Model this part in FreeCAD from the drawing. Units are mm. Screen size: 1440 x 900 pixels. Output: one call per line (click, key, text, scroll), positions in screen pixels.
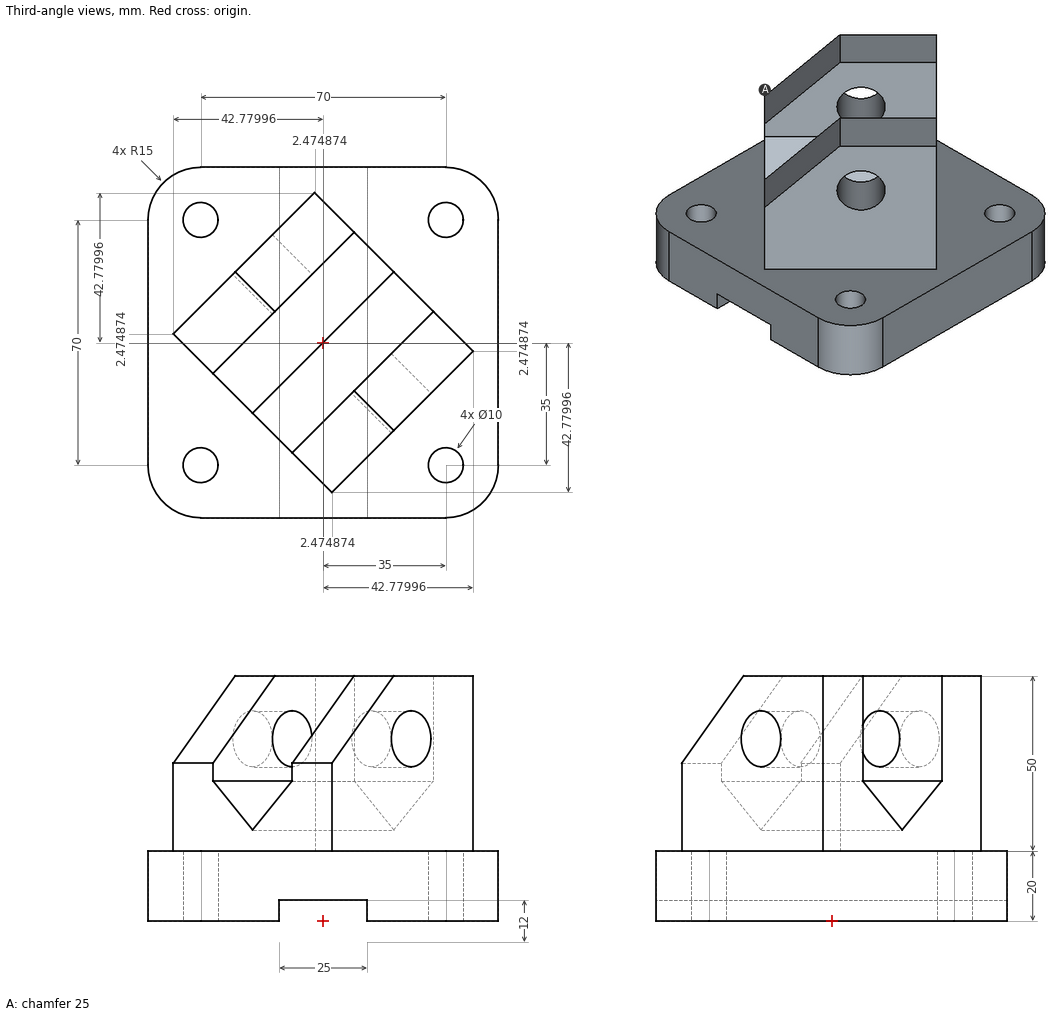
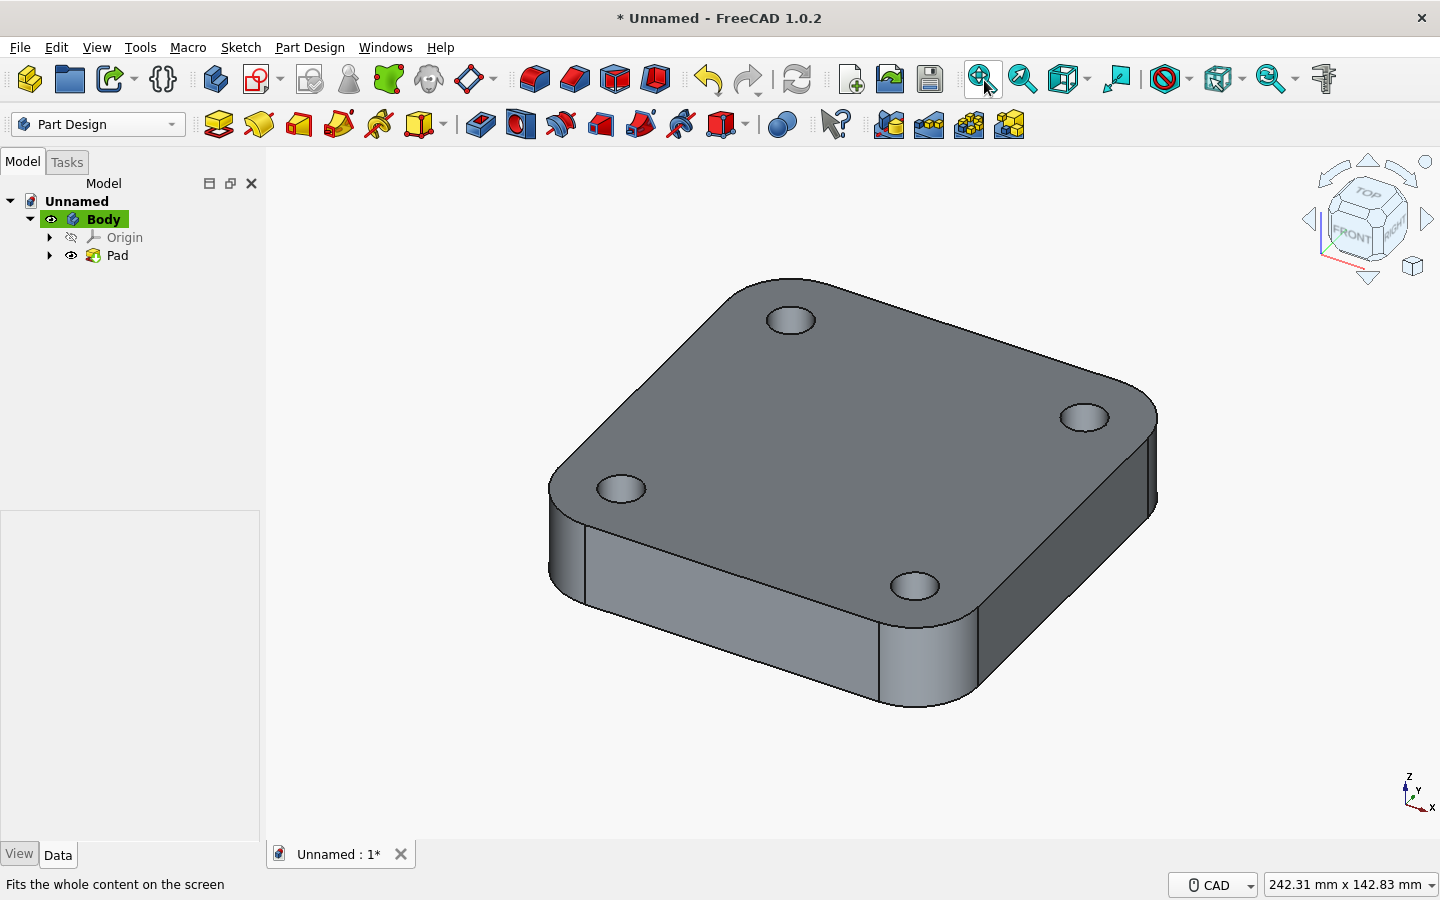
click(816, 640)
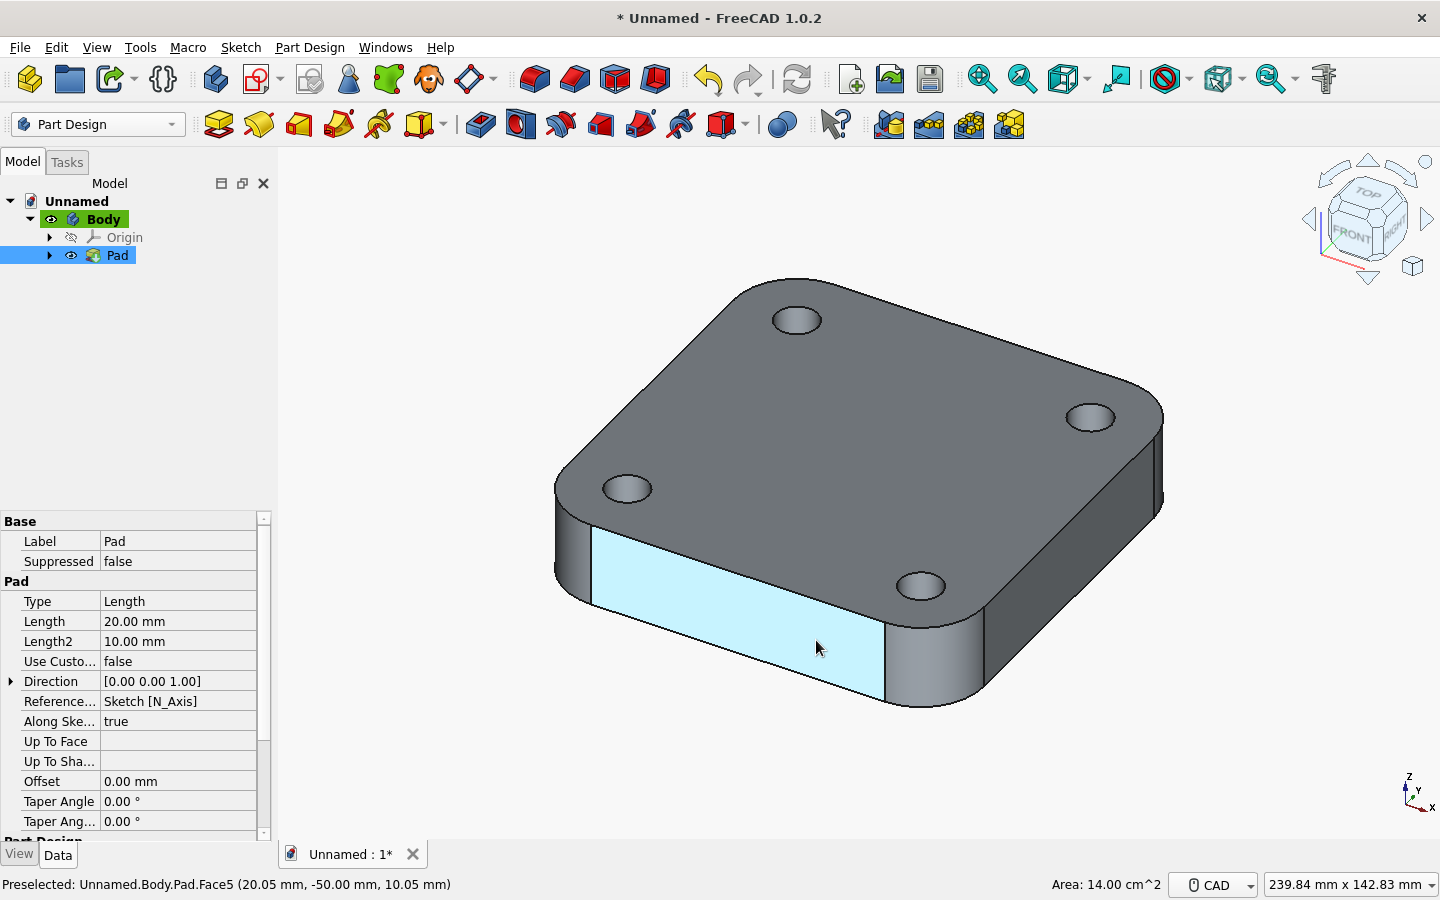
click(256, 80)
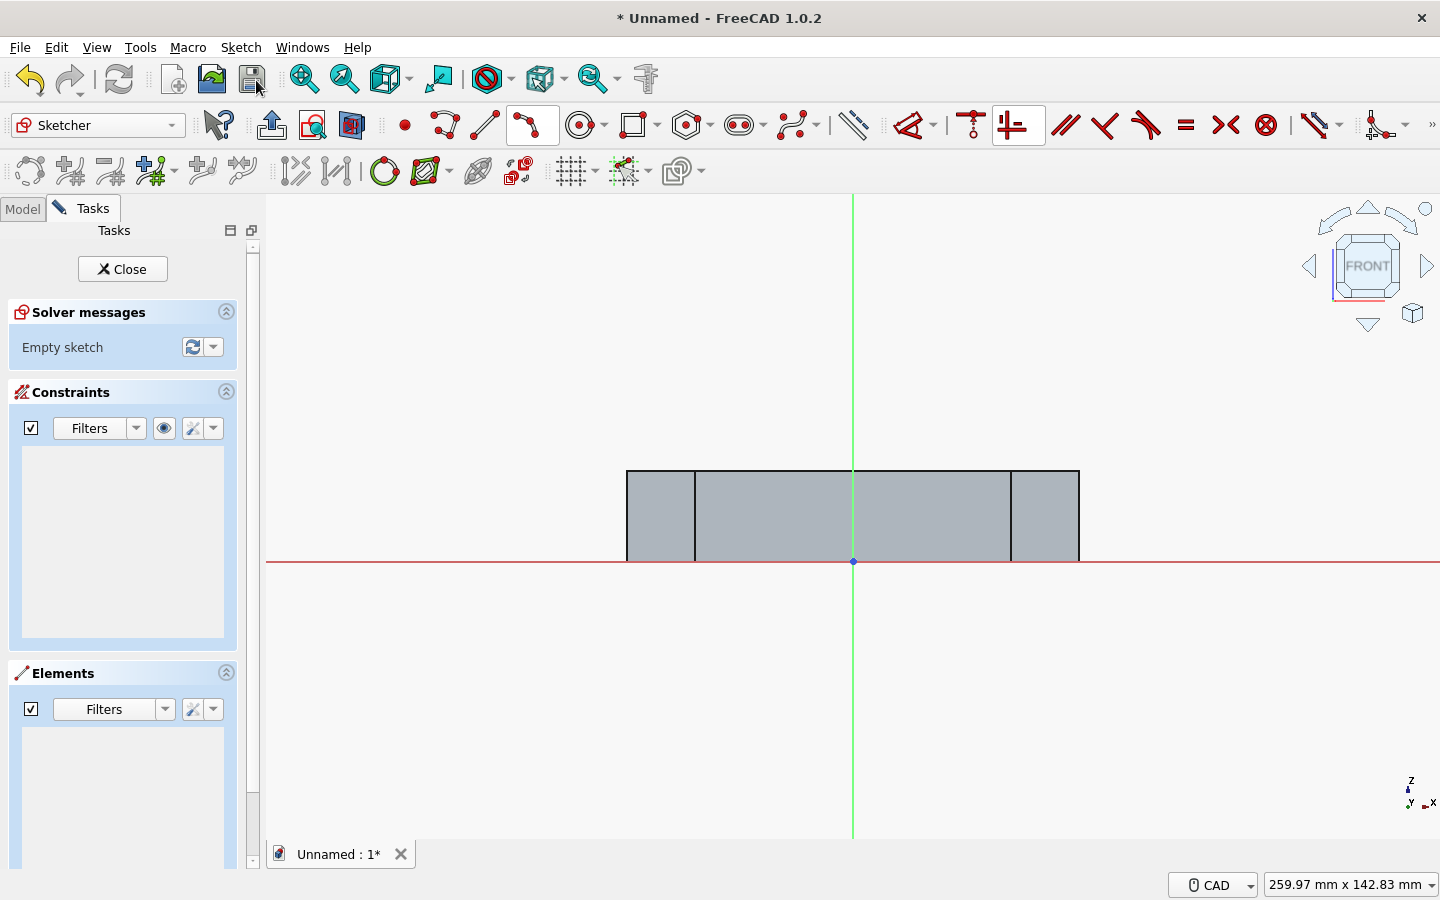
scroll(867, 571, up, 9)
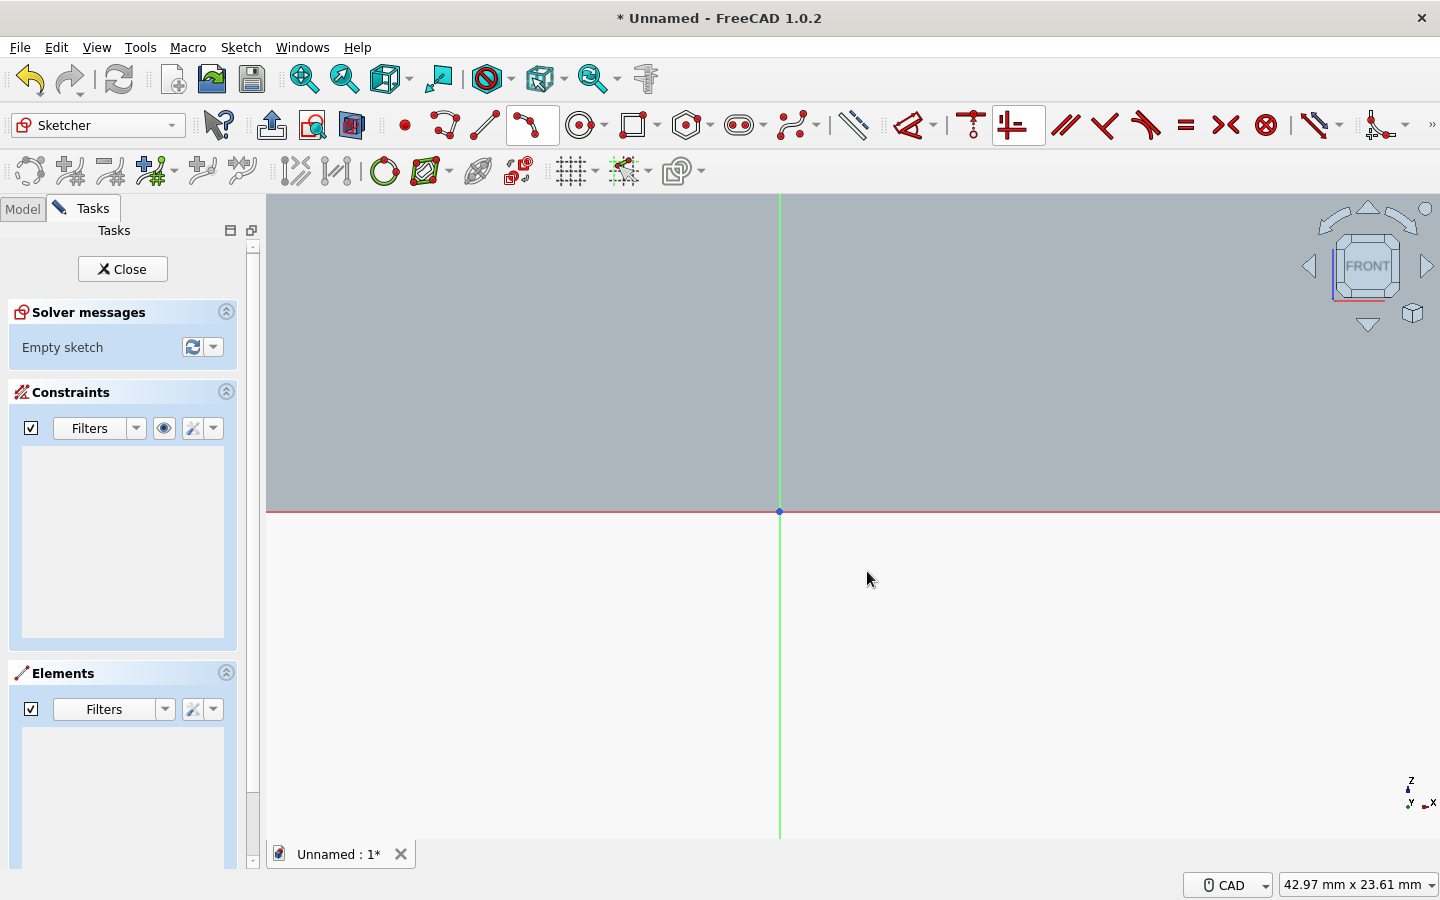
key(g)
key(v)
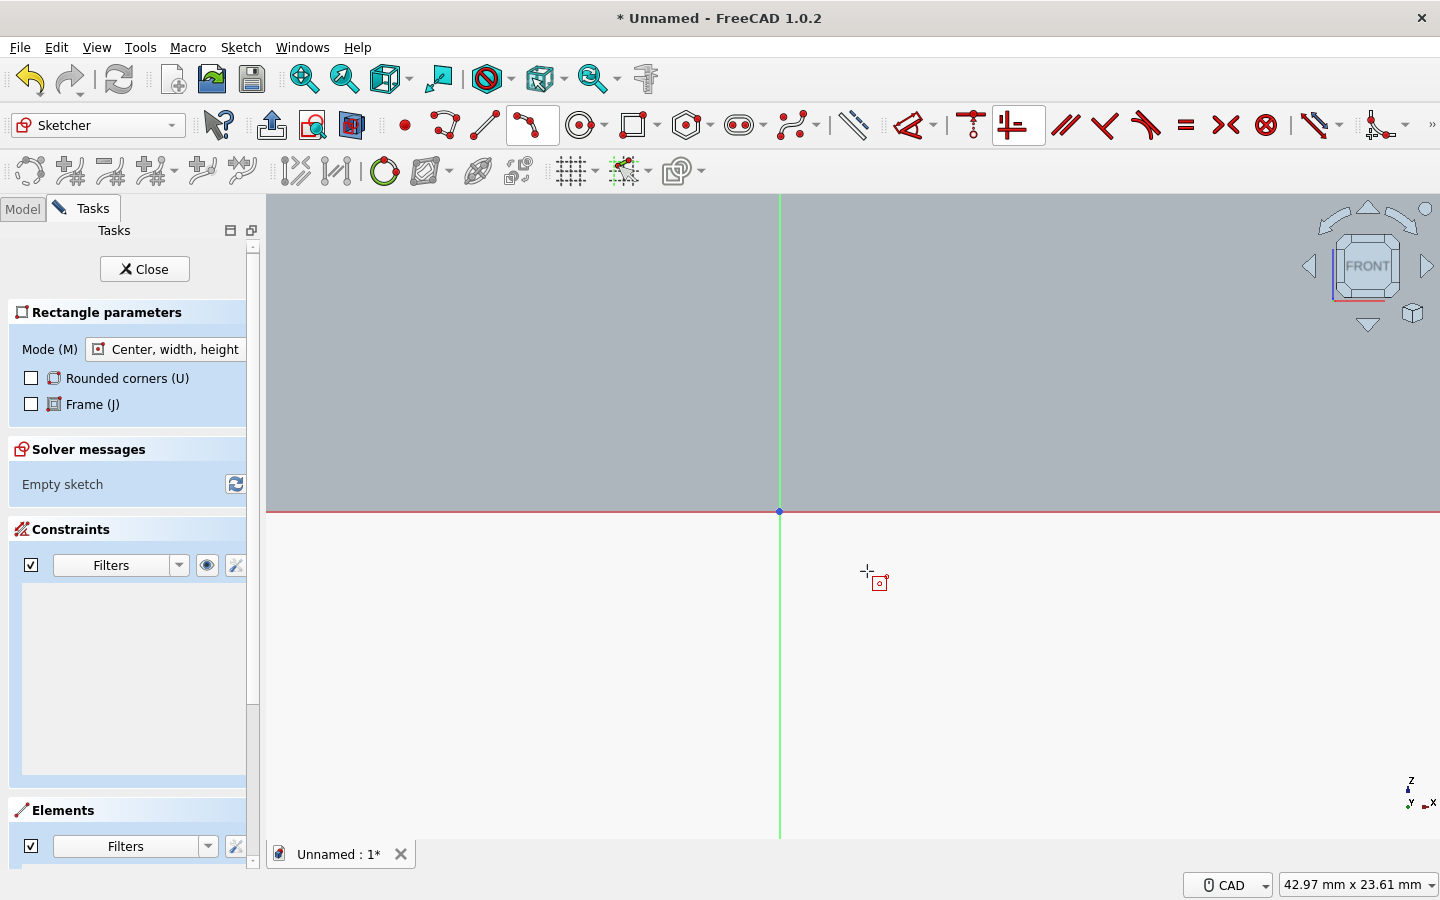
click(780, 512)
move(1121, 348)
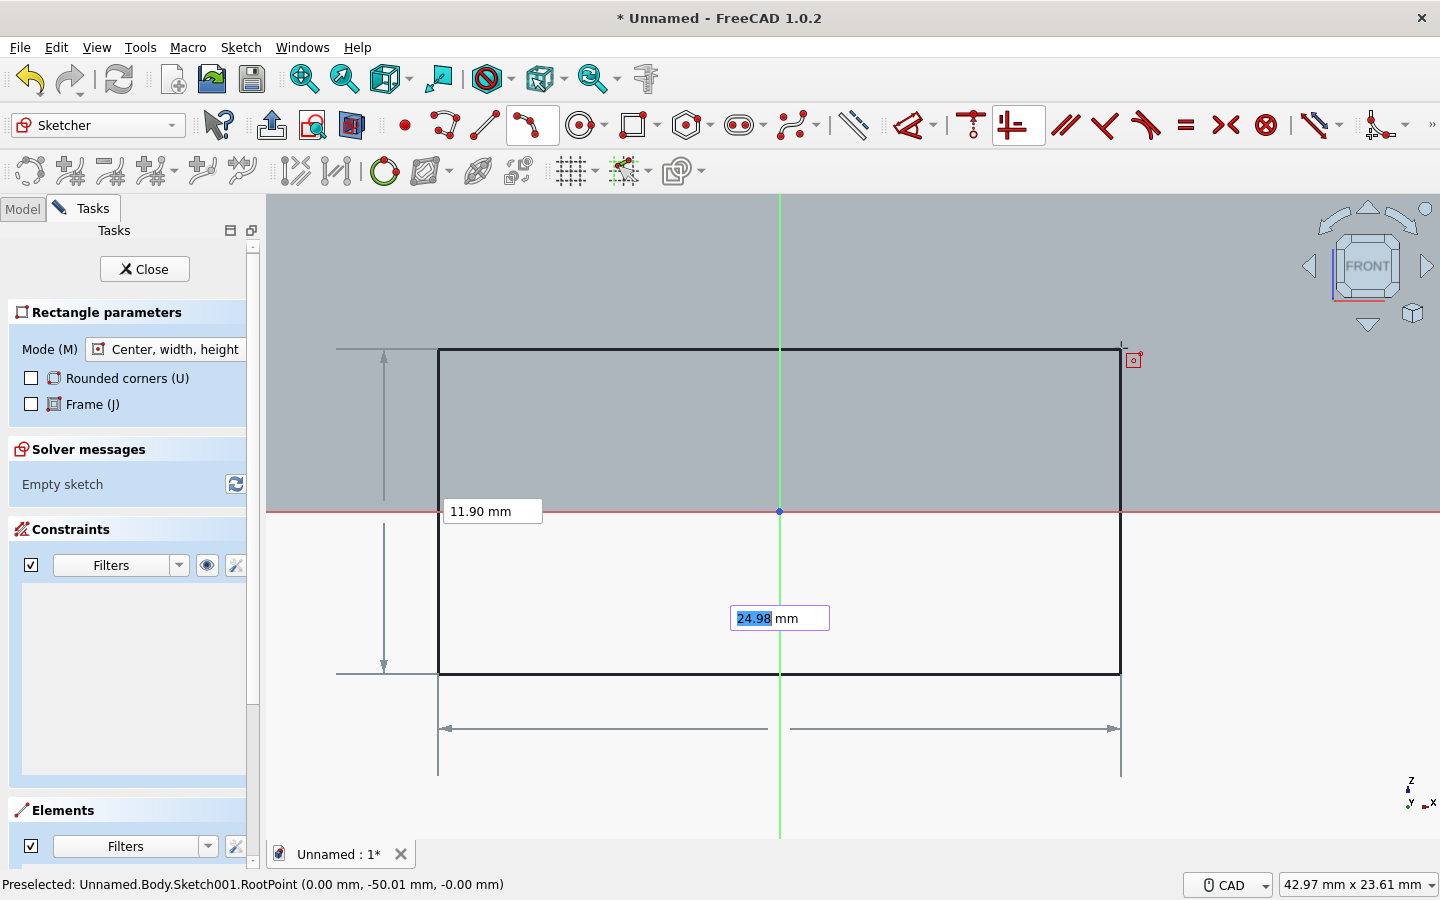
text(25)
key(Tab)
text(12)
key(Return)
key(Escape)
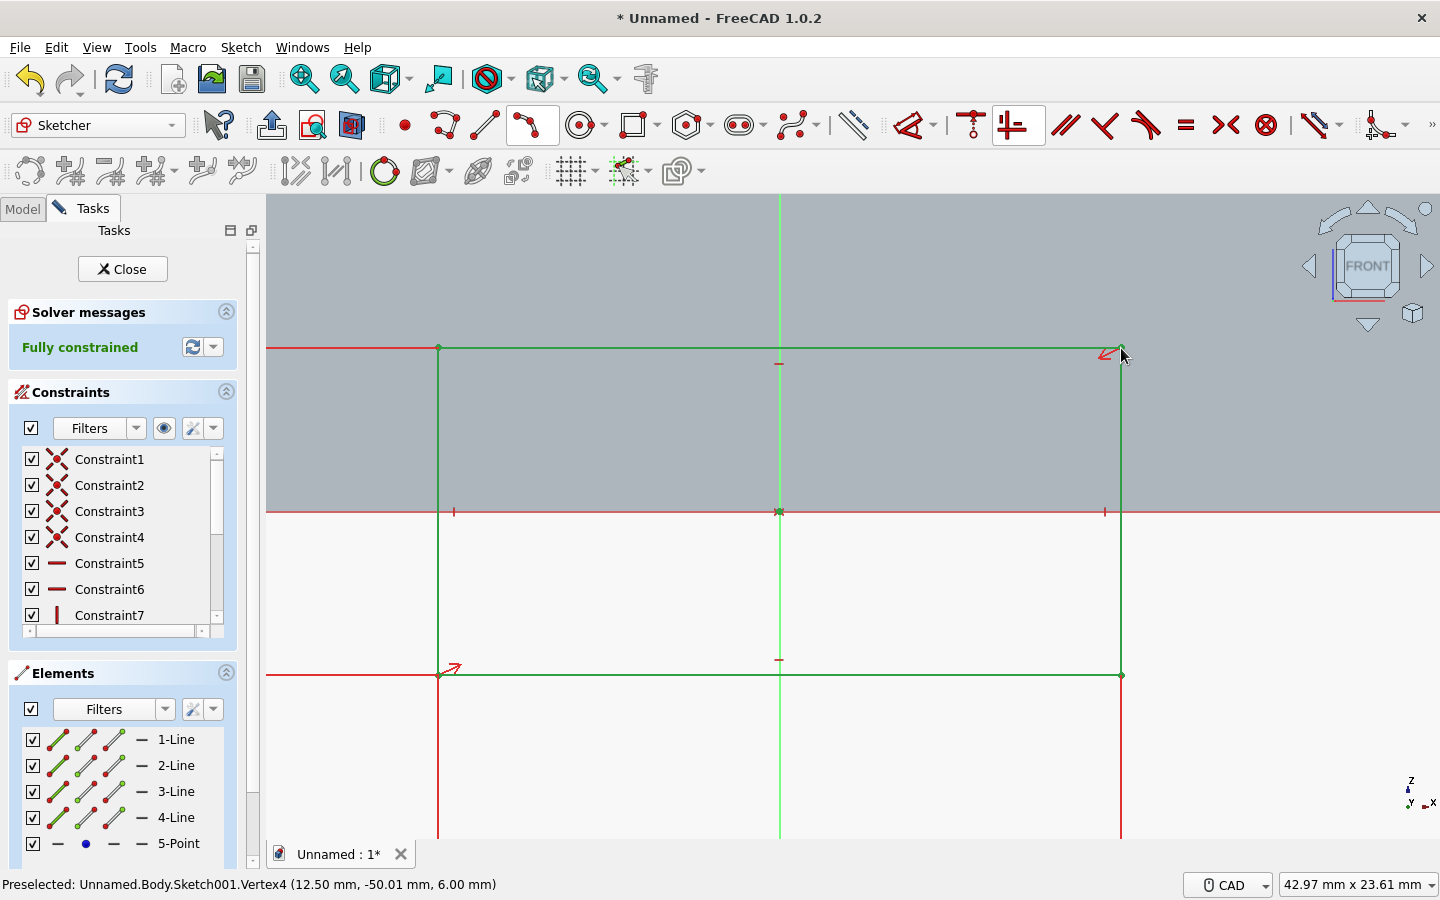
click(123, 269)